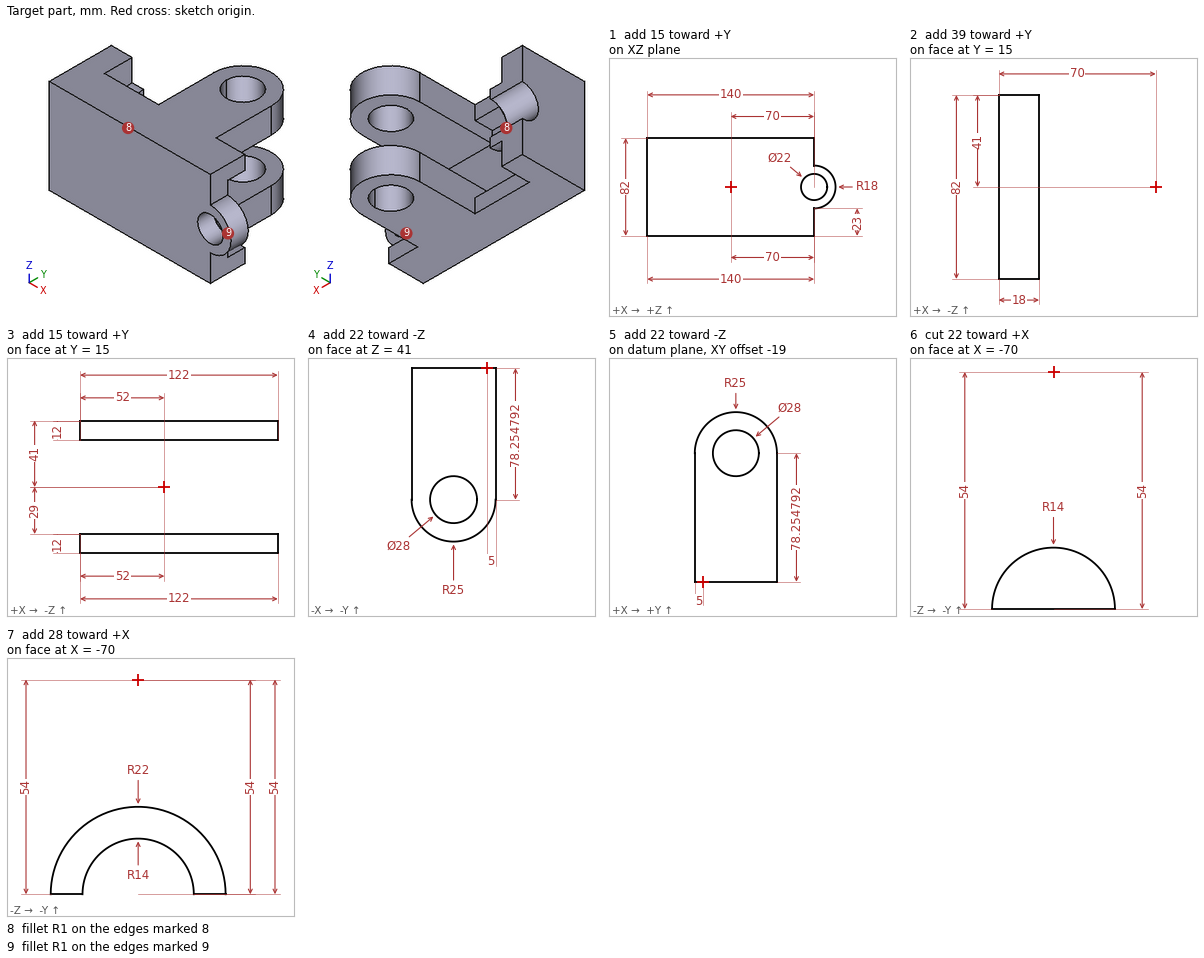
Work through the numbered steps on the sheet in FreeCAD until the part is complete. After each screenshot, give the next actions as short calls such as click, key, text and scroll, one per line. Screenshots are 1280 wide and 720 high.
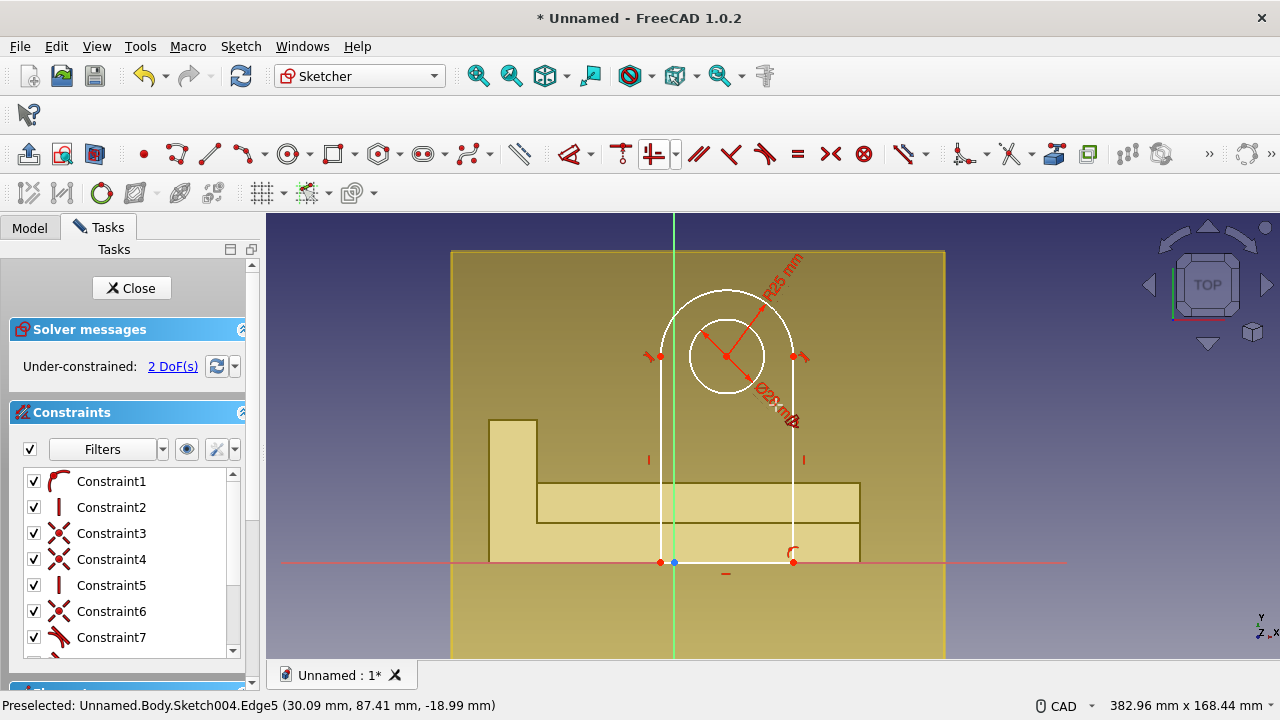
scroll(661, 563, up, 6)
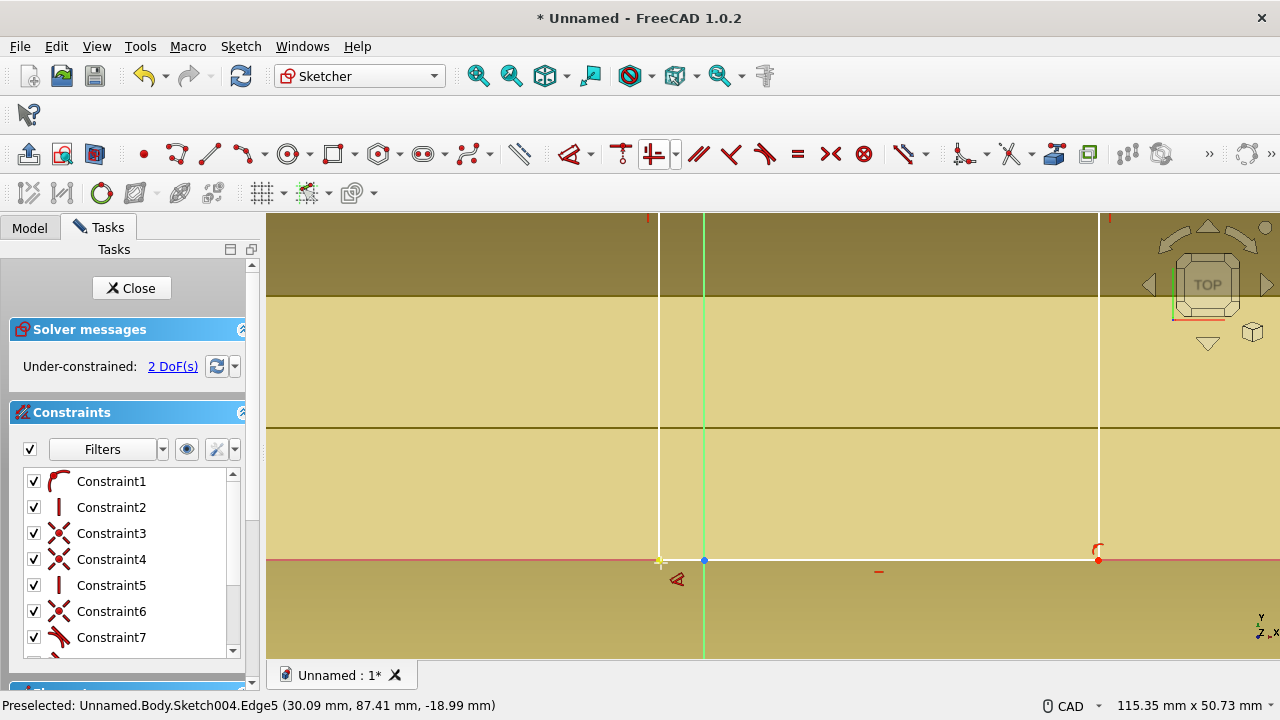
click(659, 560)
click(682, 594)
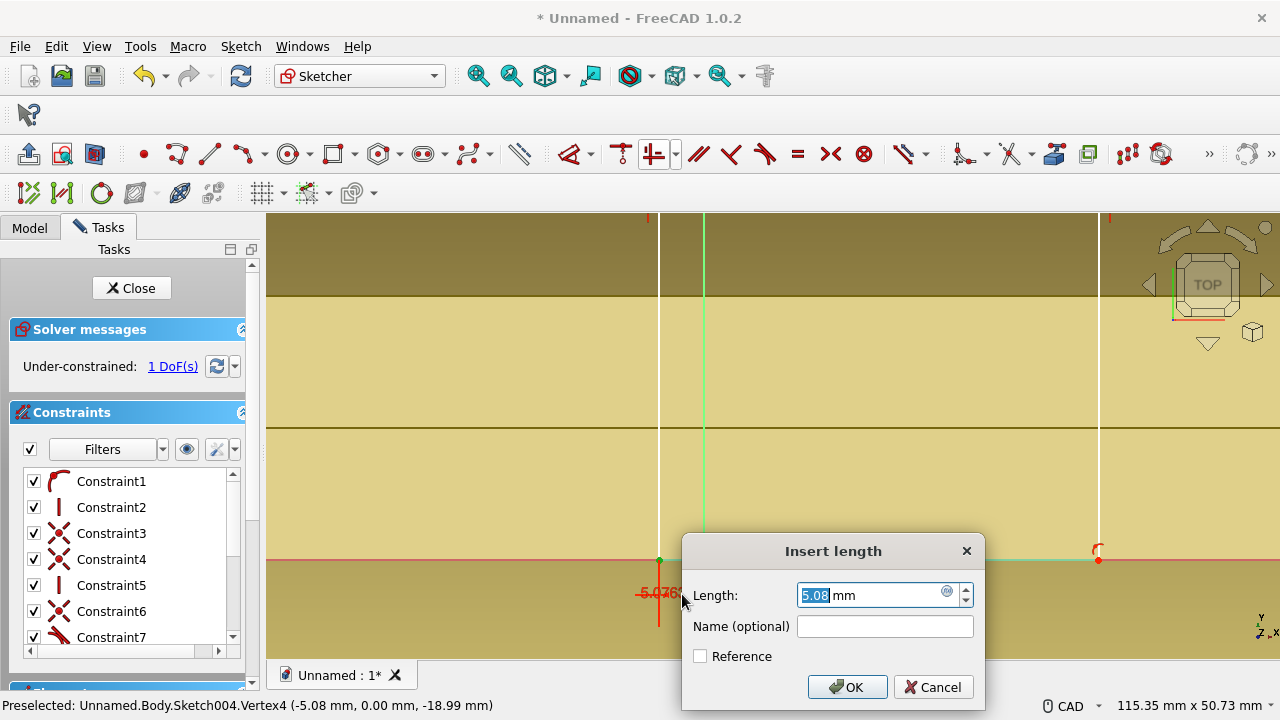
text(5)
key(Return)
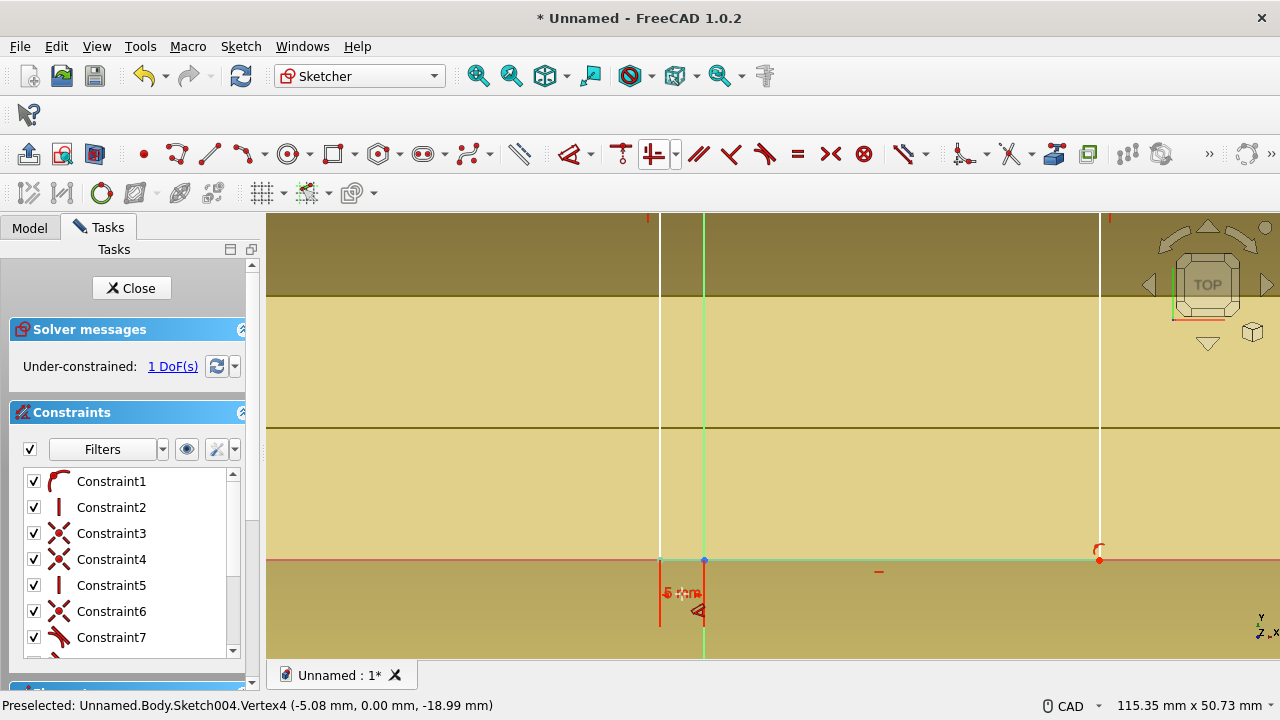
scroll(629, 578, down, 6)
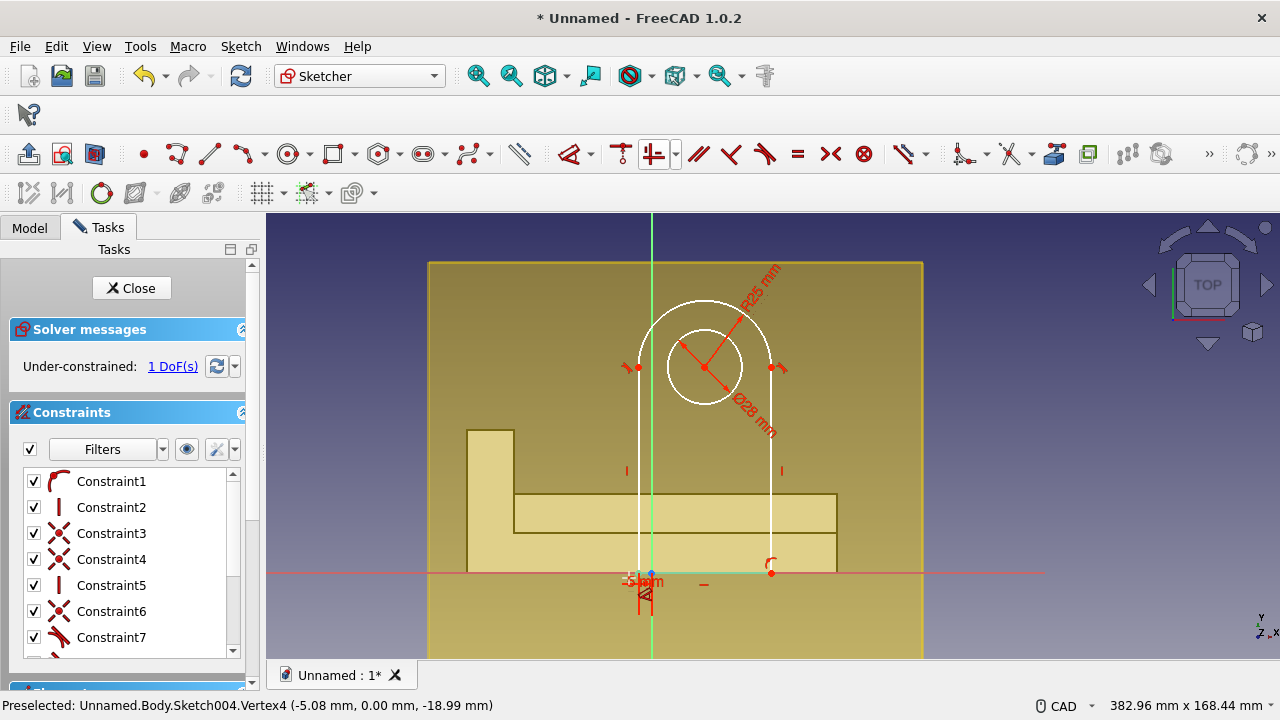
click(771, 511)
click(805, 470)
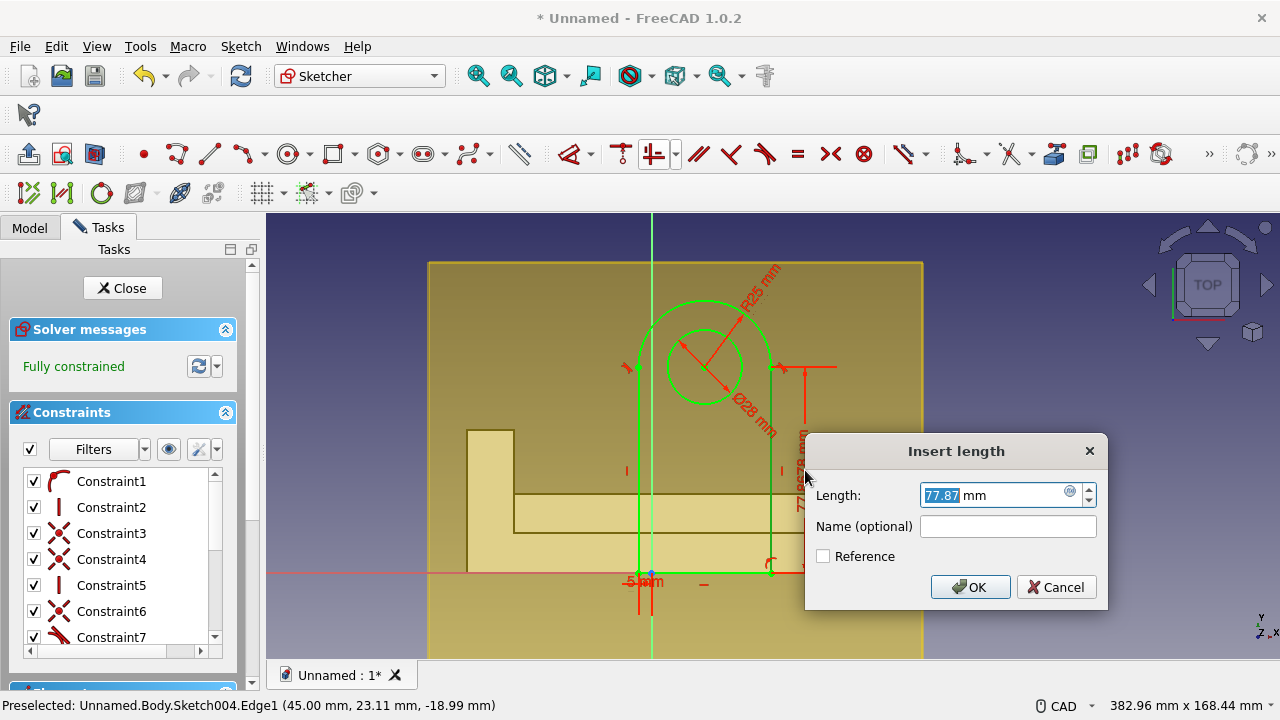
text(78.254792)
key(Return)
key(Escape)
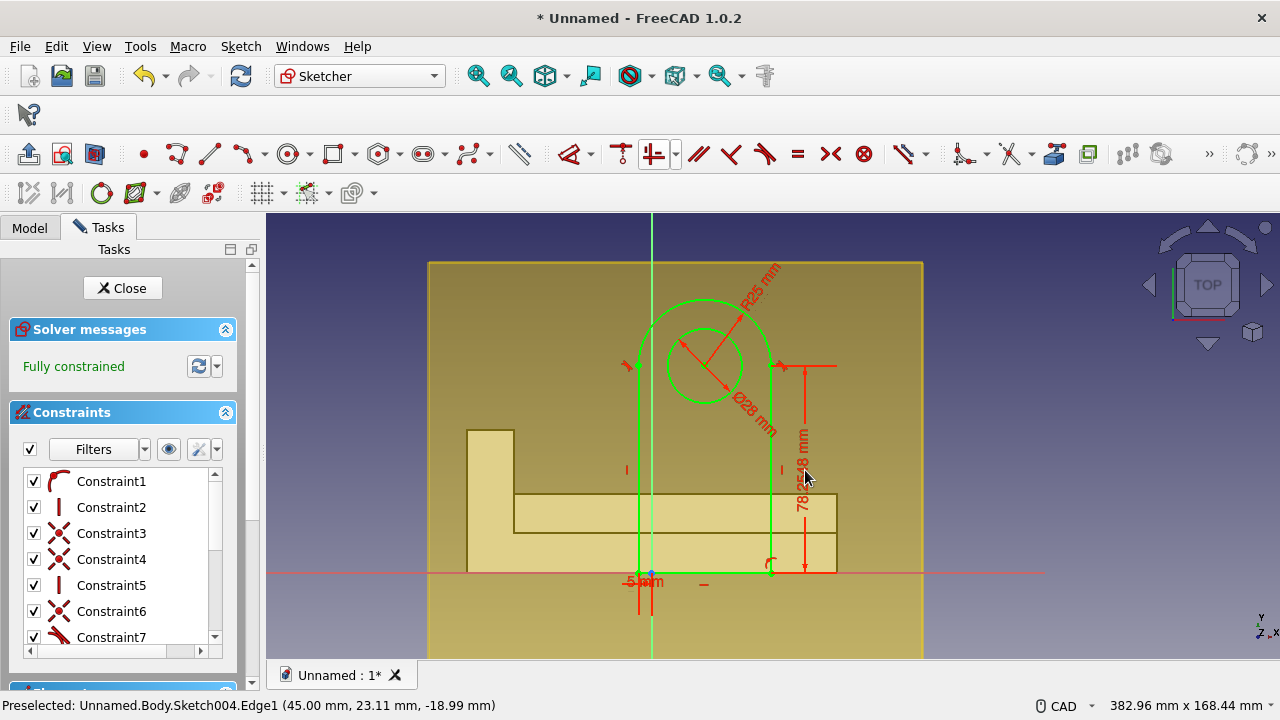
click(123, 288)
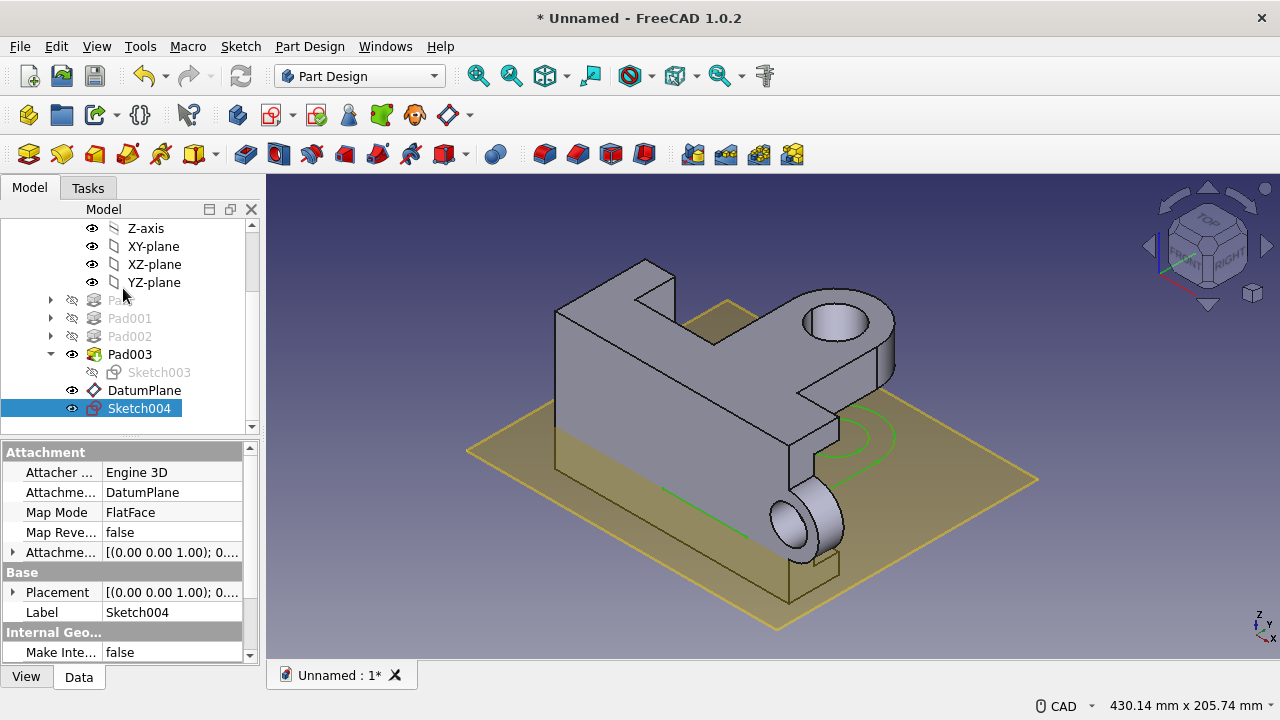
click(29, 154)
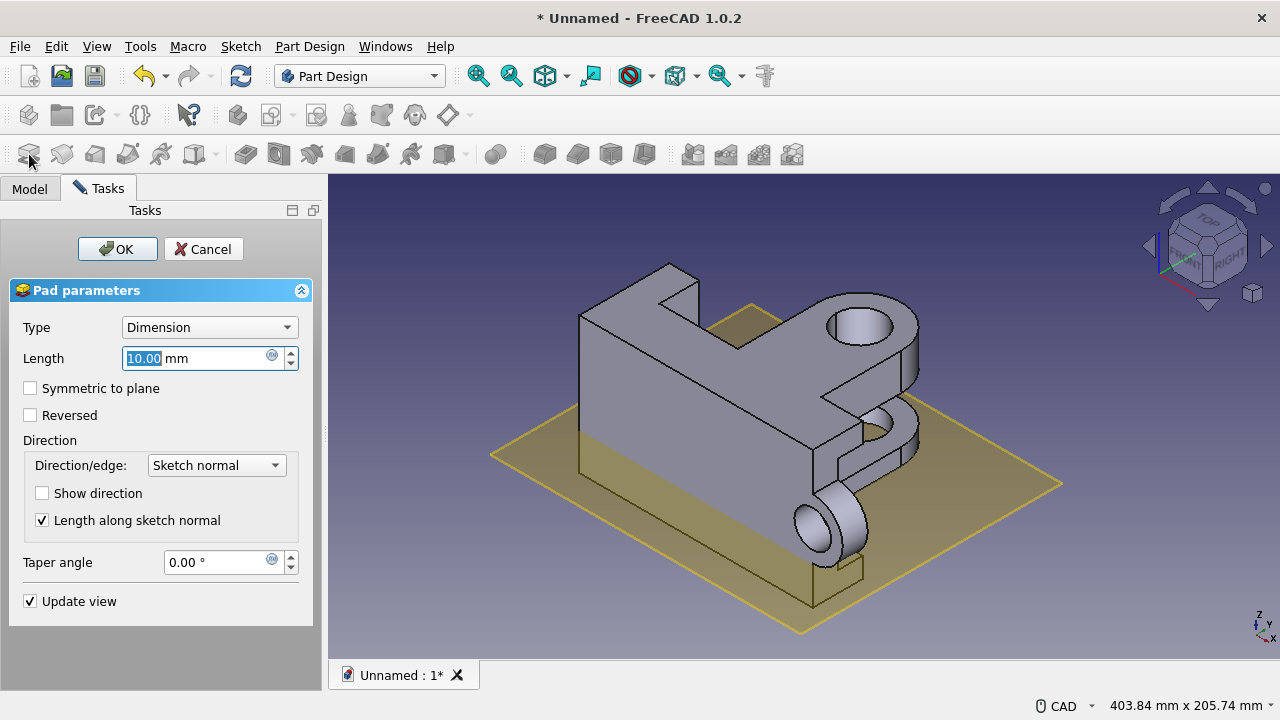
text(22)
key(Tab)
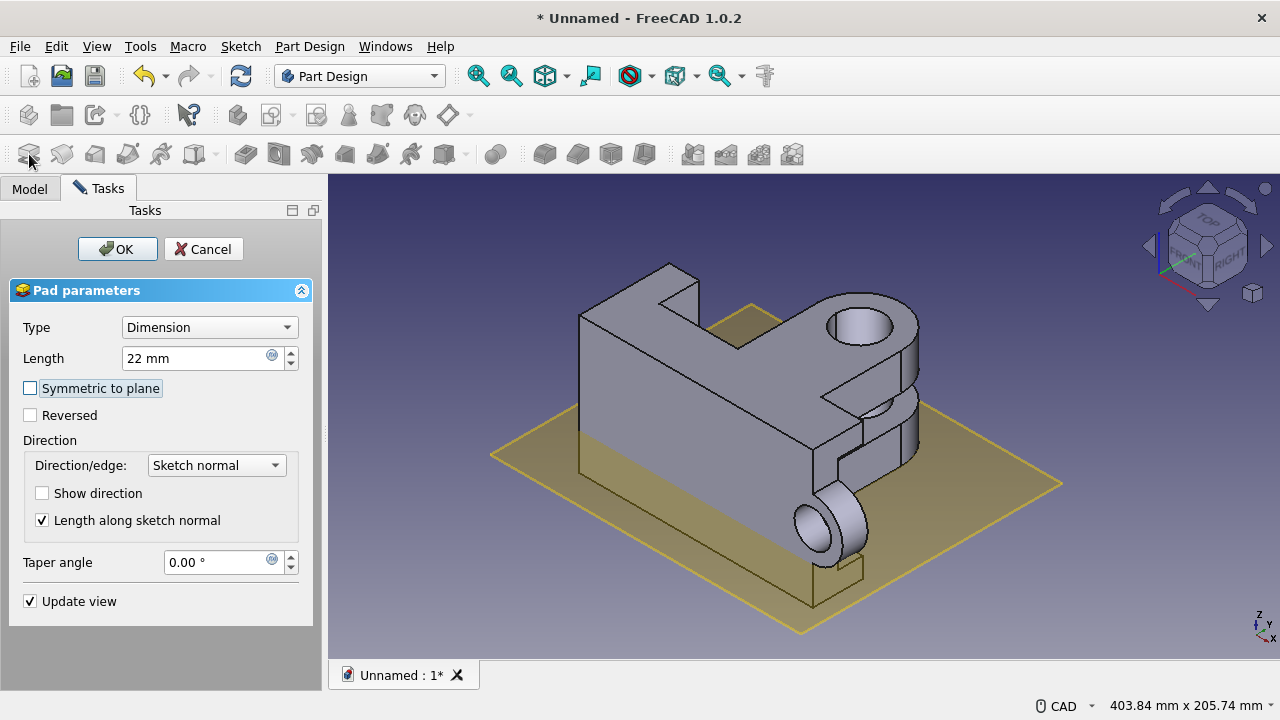
click(31, 415)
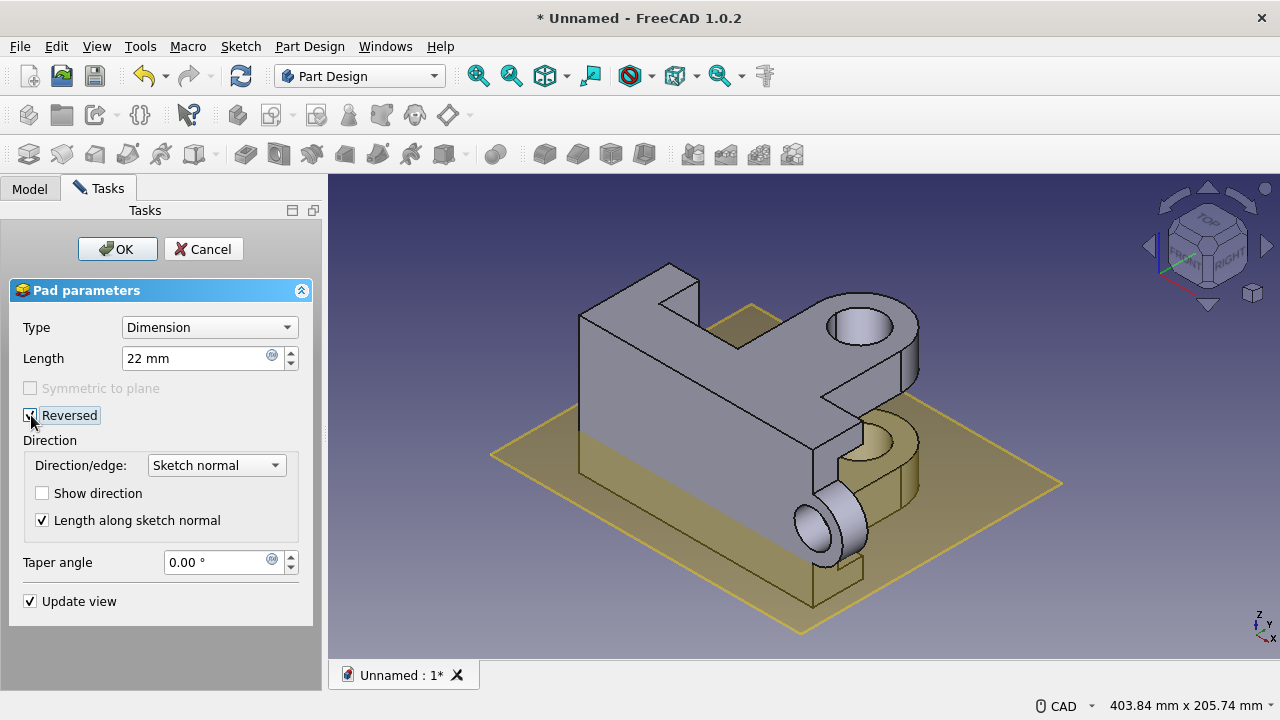
click(118, 249)